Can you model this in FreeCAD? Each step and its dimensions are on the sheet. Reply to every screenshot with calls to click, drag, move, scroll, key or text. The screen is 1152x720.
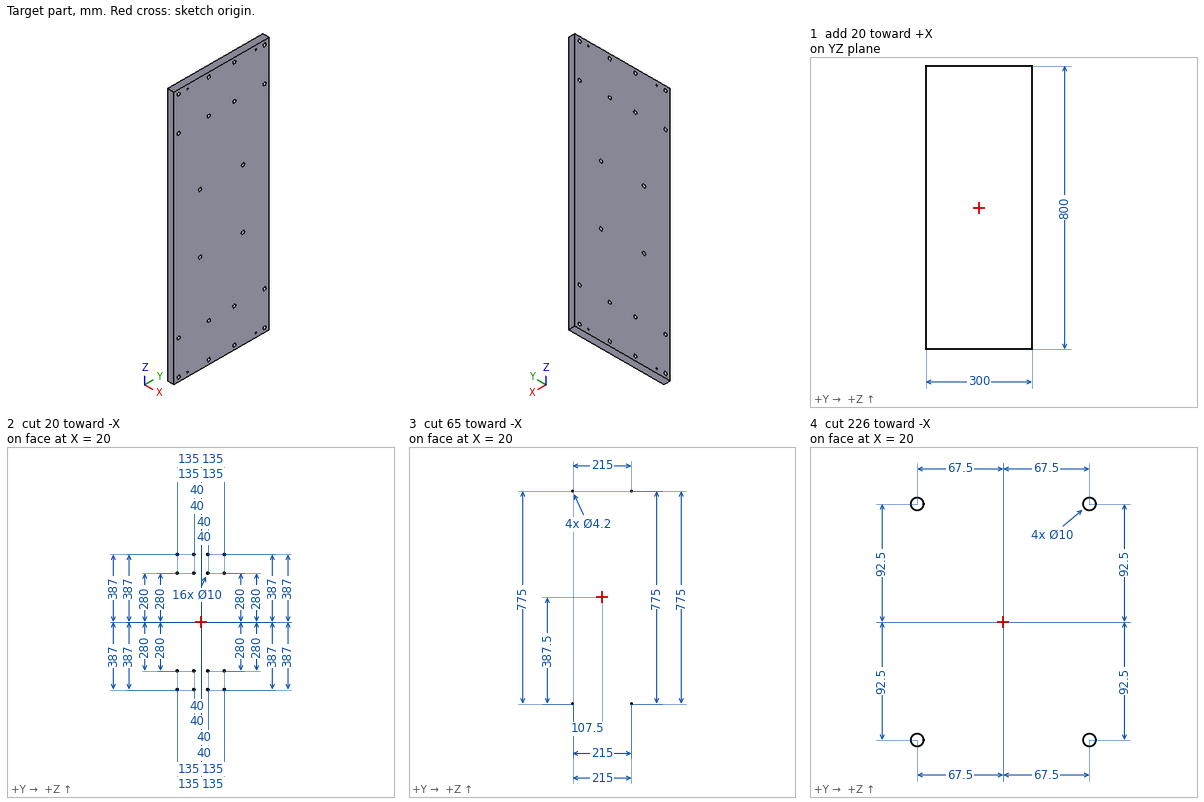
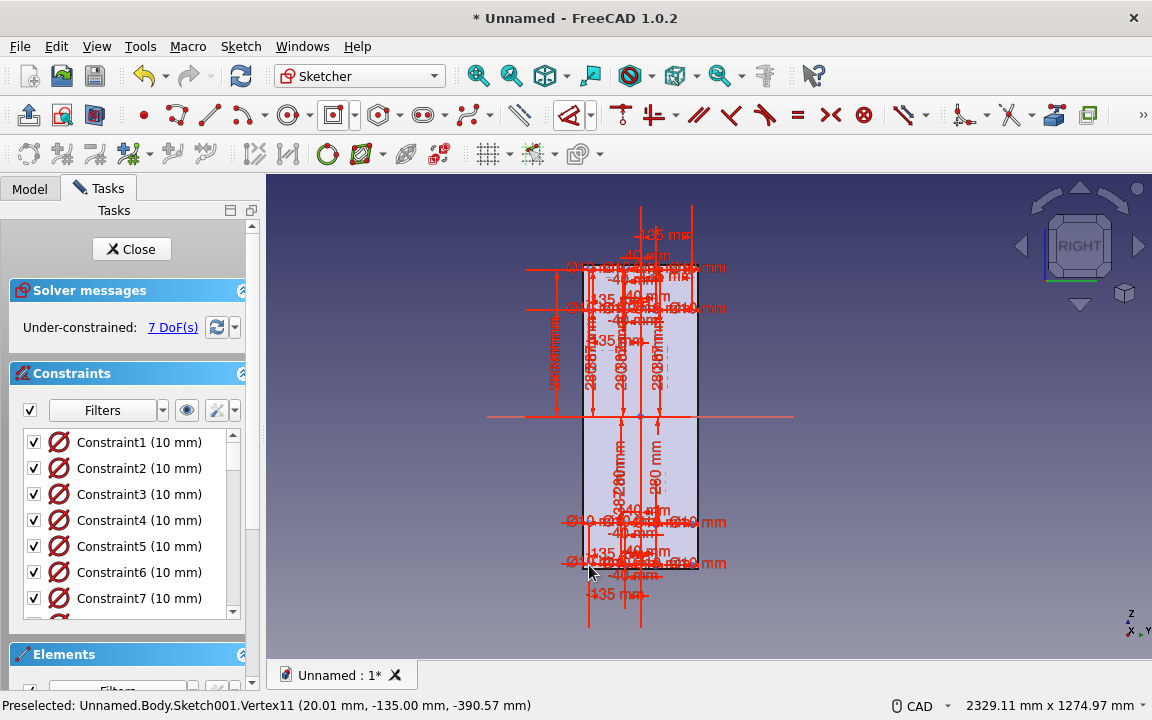
click(625, 565)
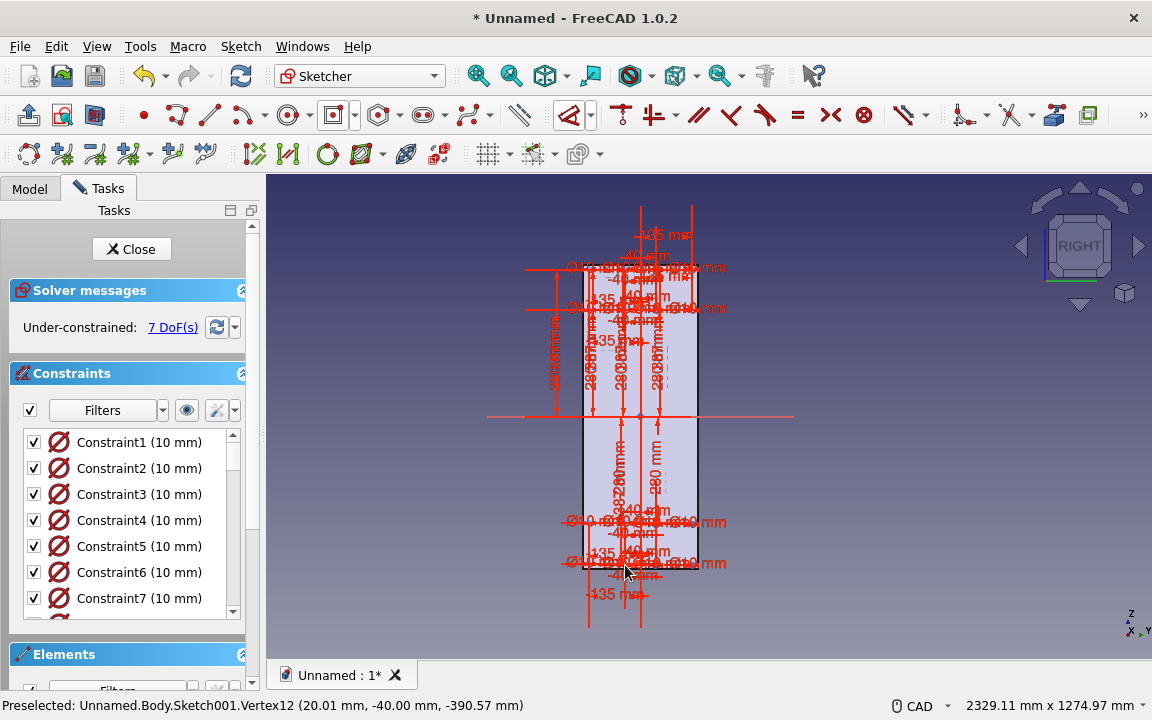
key(i)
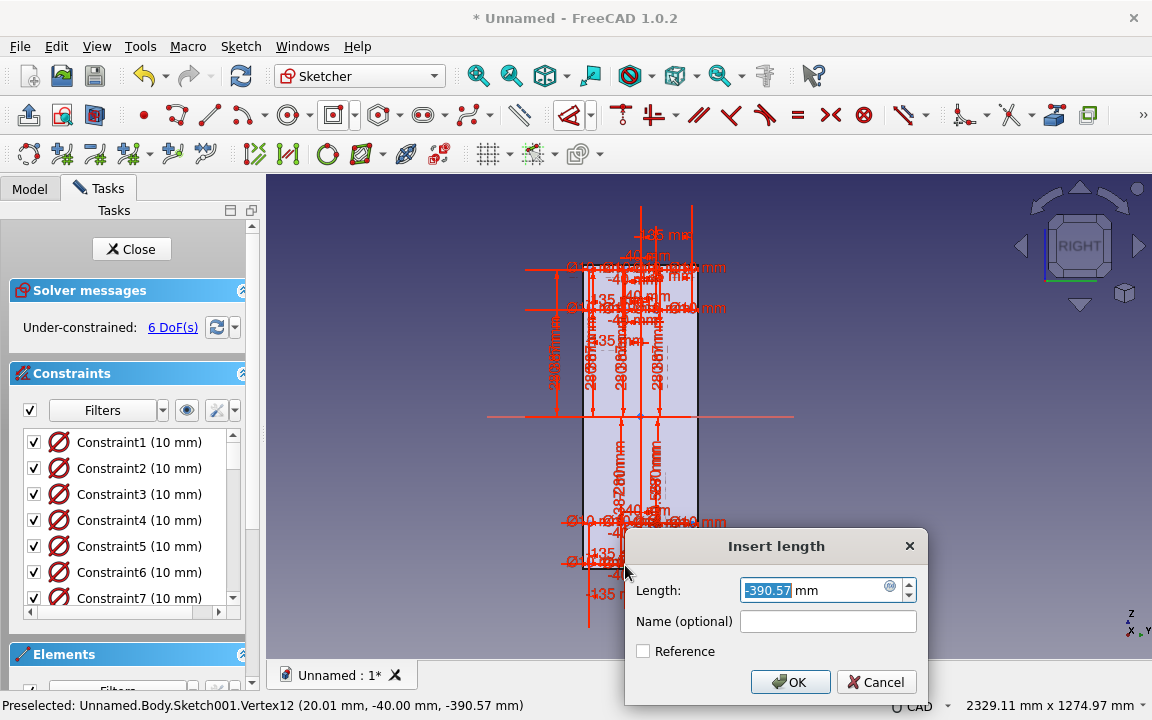
text(-387)
key(Return)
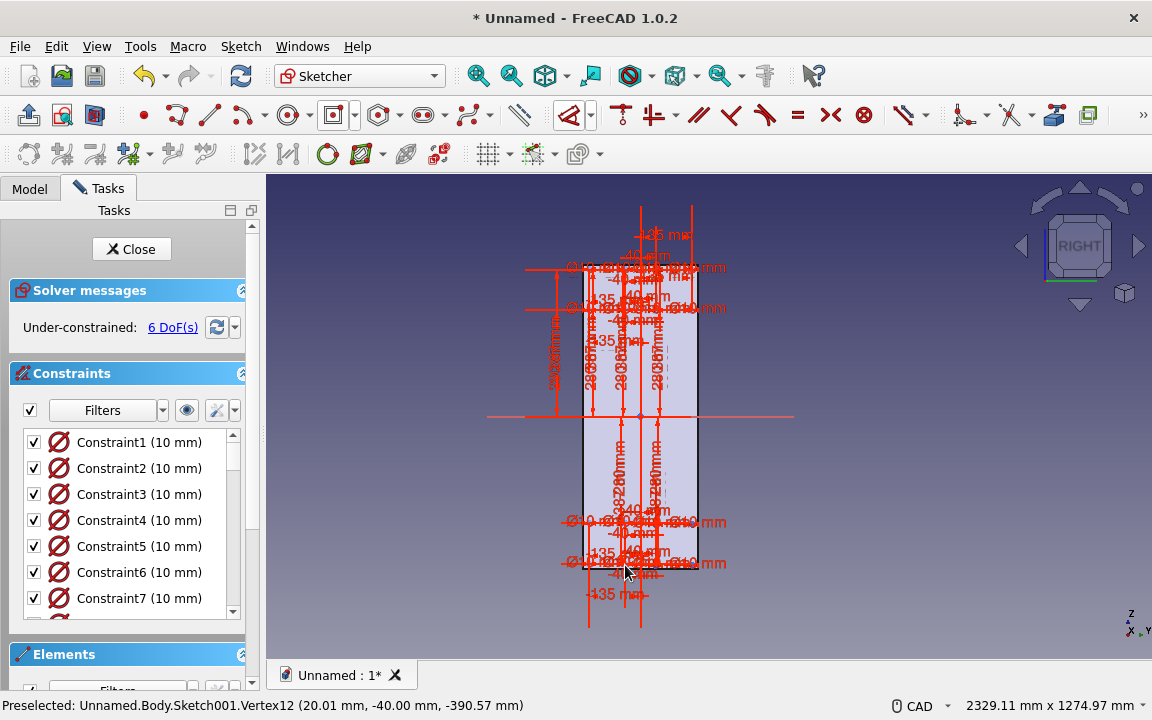
click(692, 524)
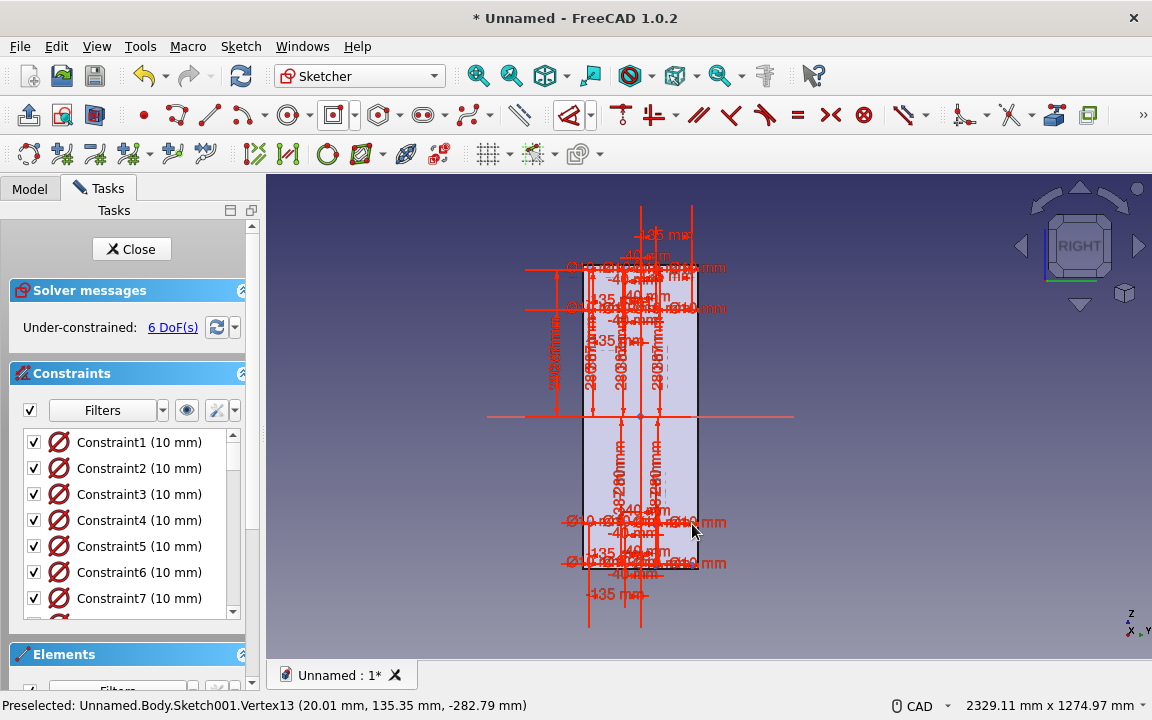
key(l)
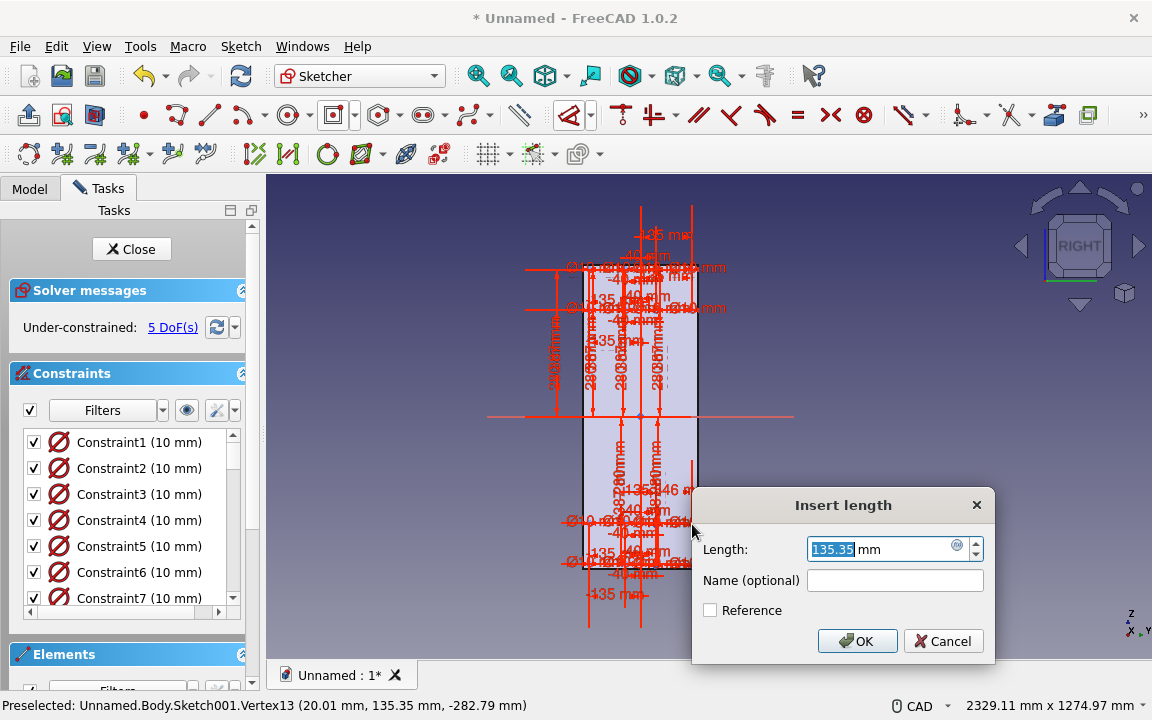
text(135)
key(Return)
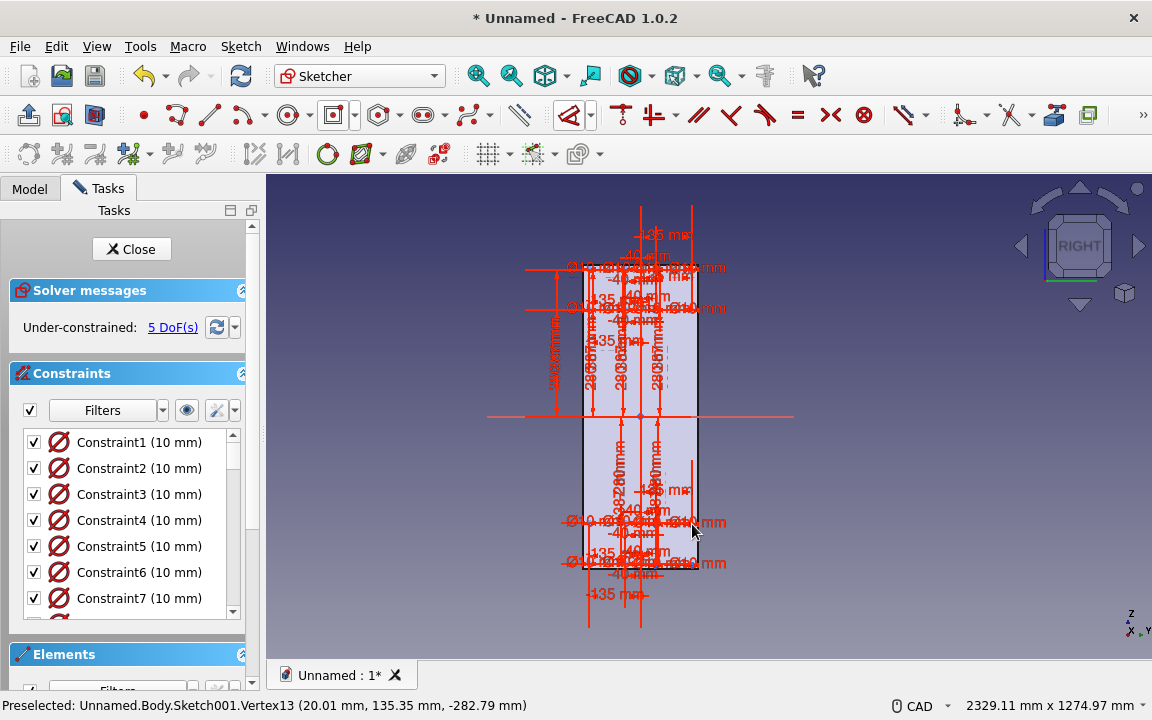
click(692, 524)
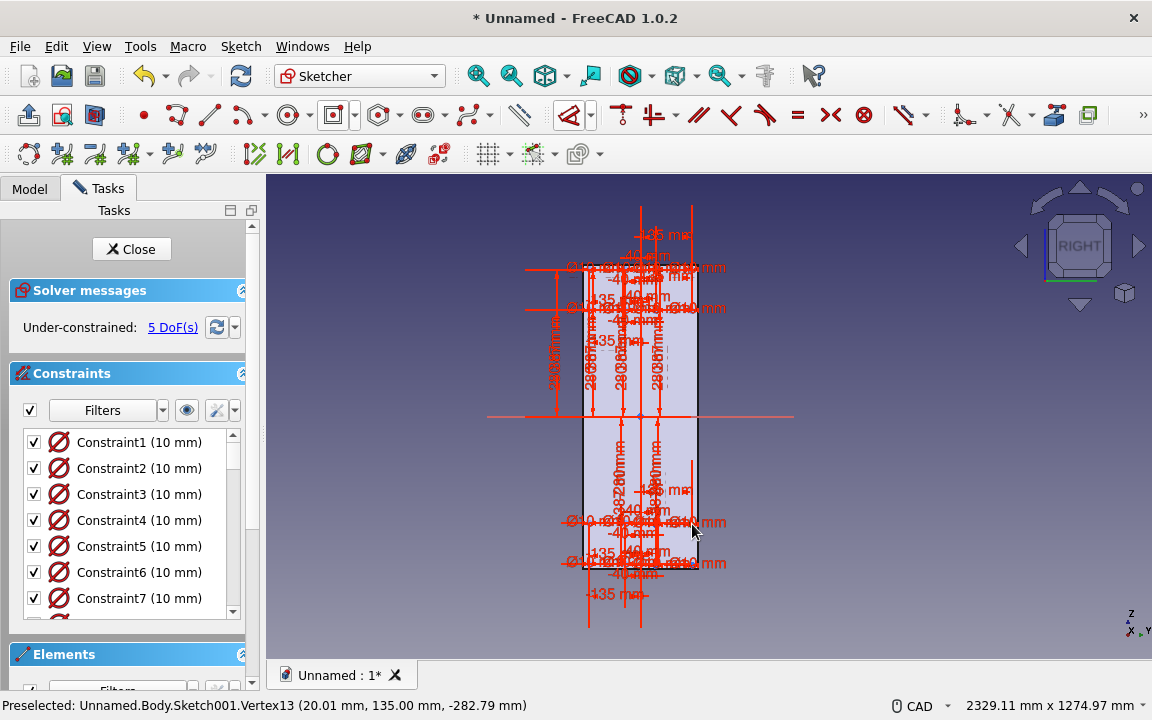
click(590, 116)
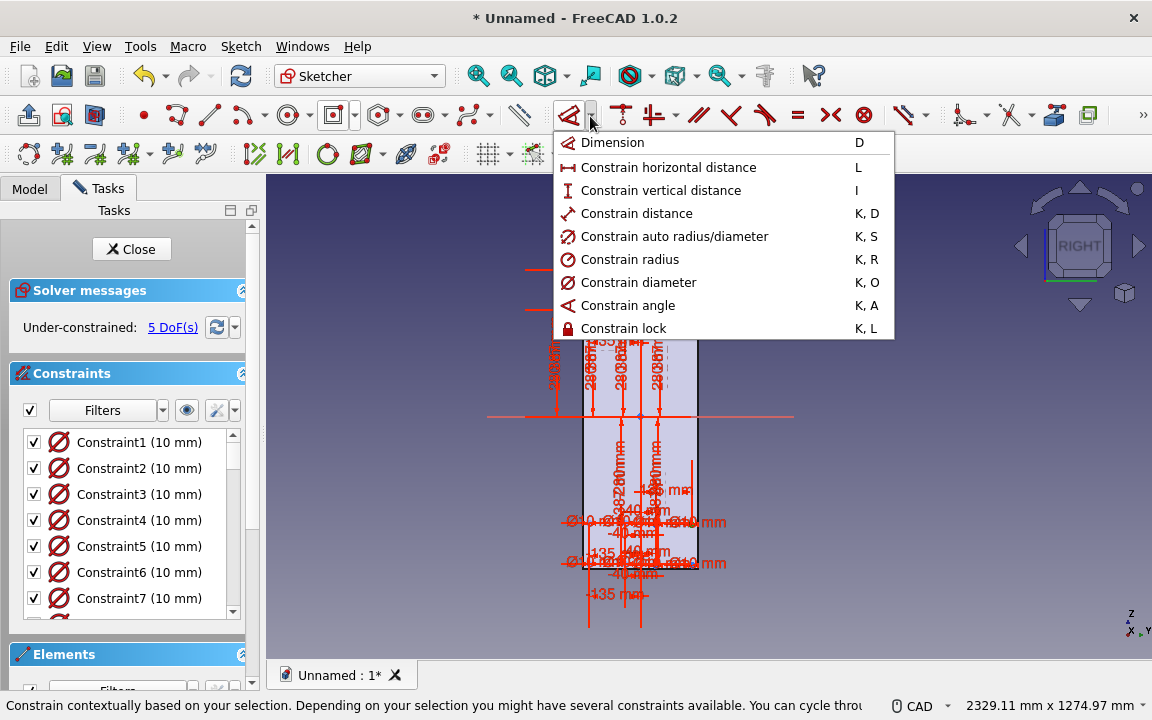
click(724, 190)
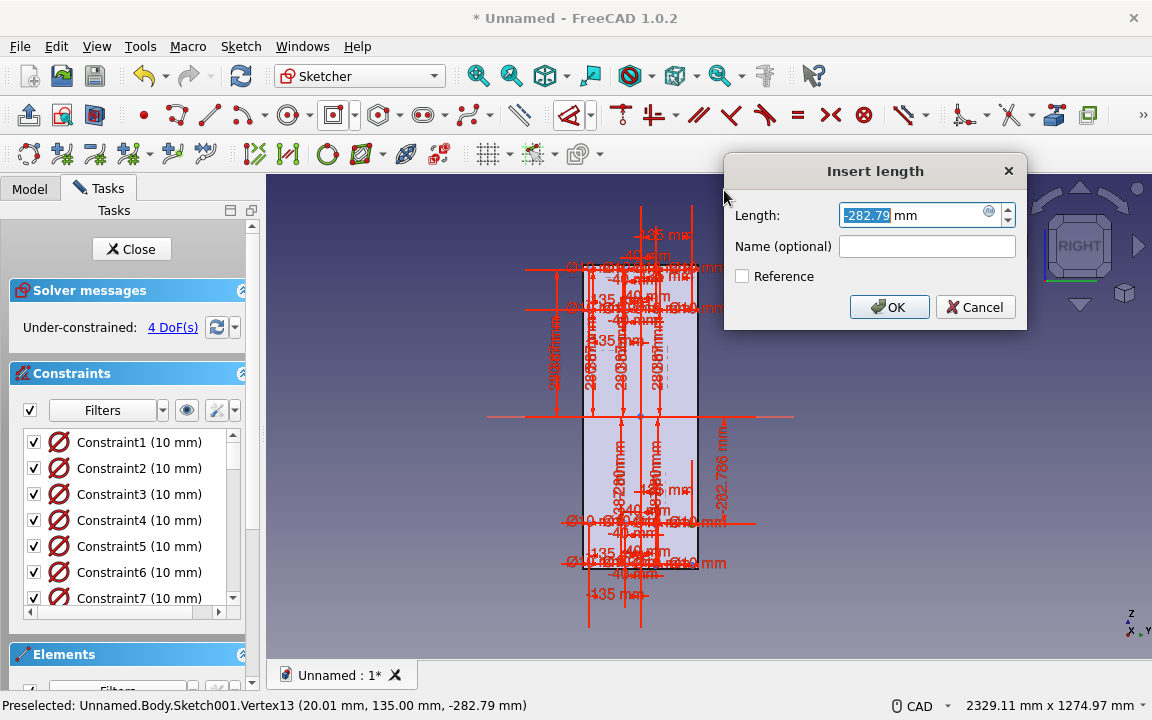
text(-280)
key(Return)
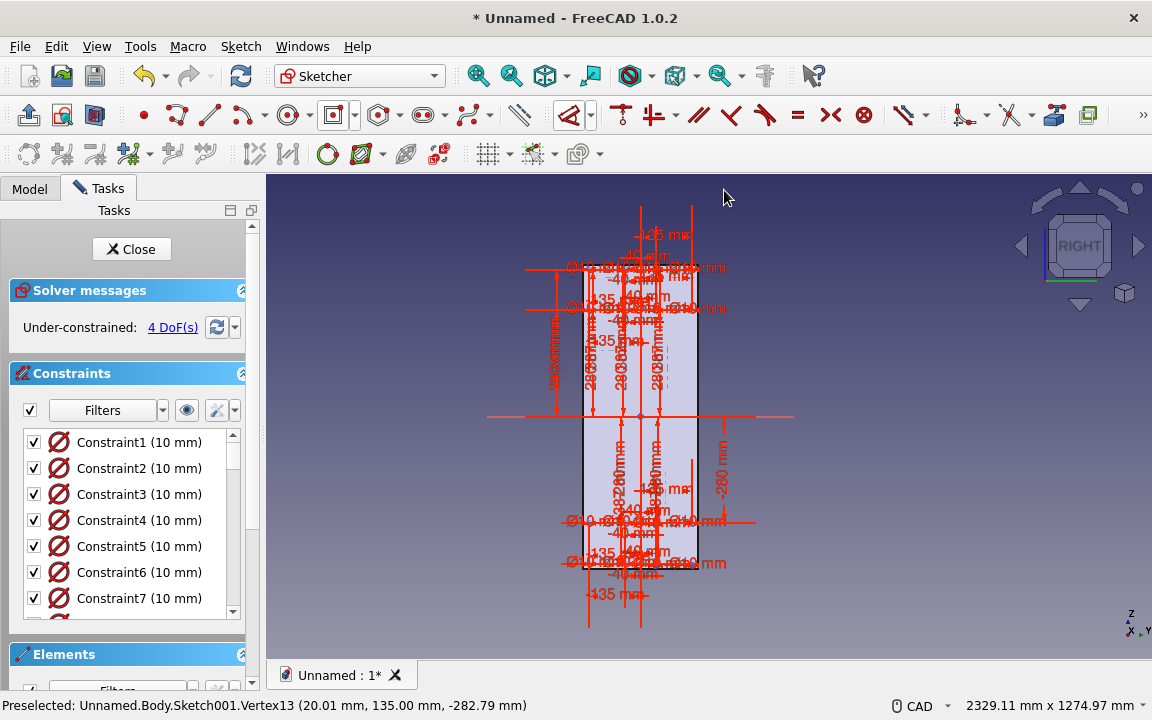
click(692, 565)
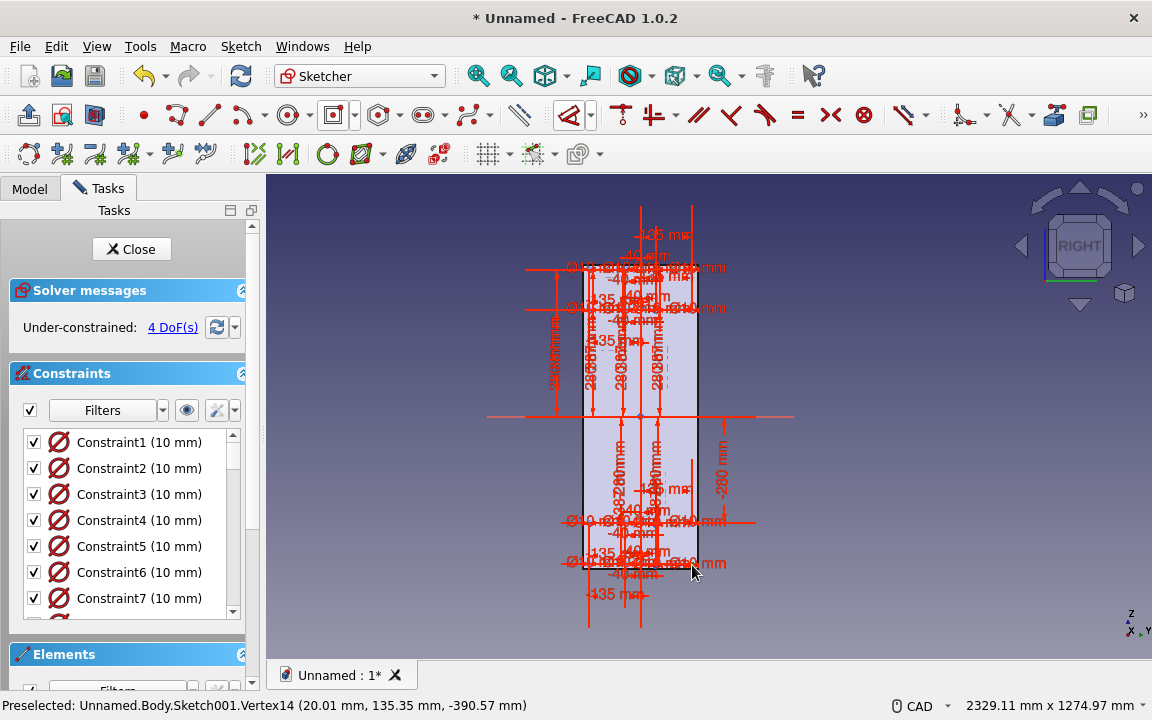
key(l)